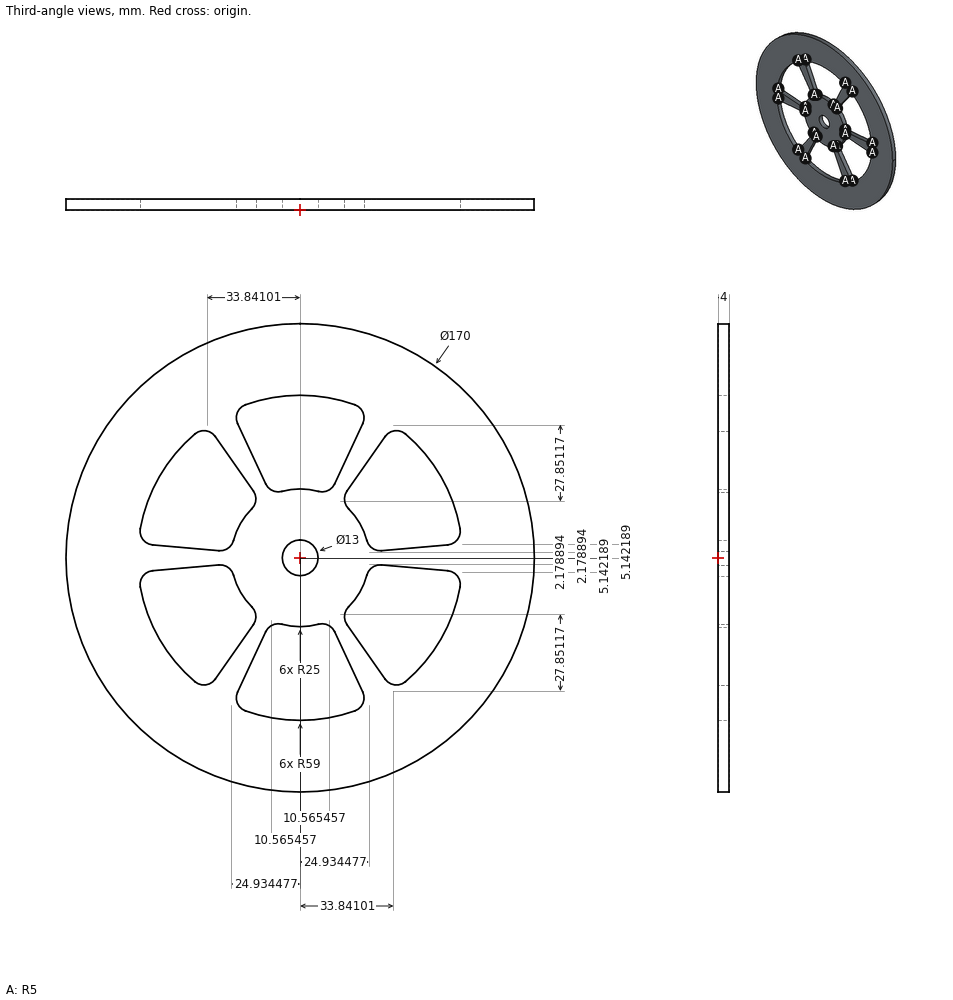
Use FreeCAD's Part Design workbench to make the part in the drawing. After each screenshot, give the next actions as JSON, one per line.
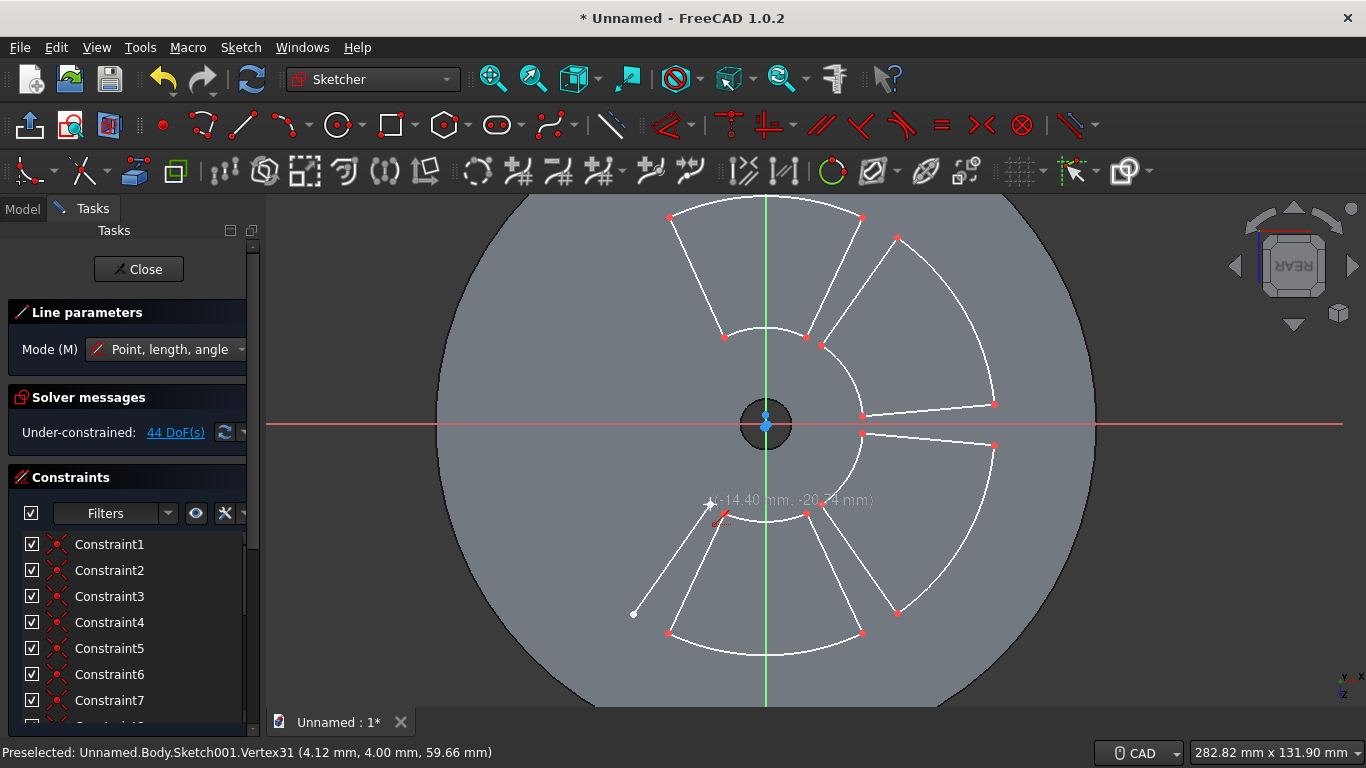
{"action": "scroll", "coordinate": [669, 433], "scroll_direction": "up", "scroll_amount": 4}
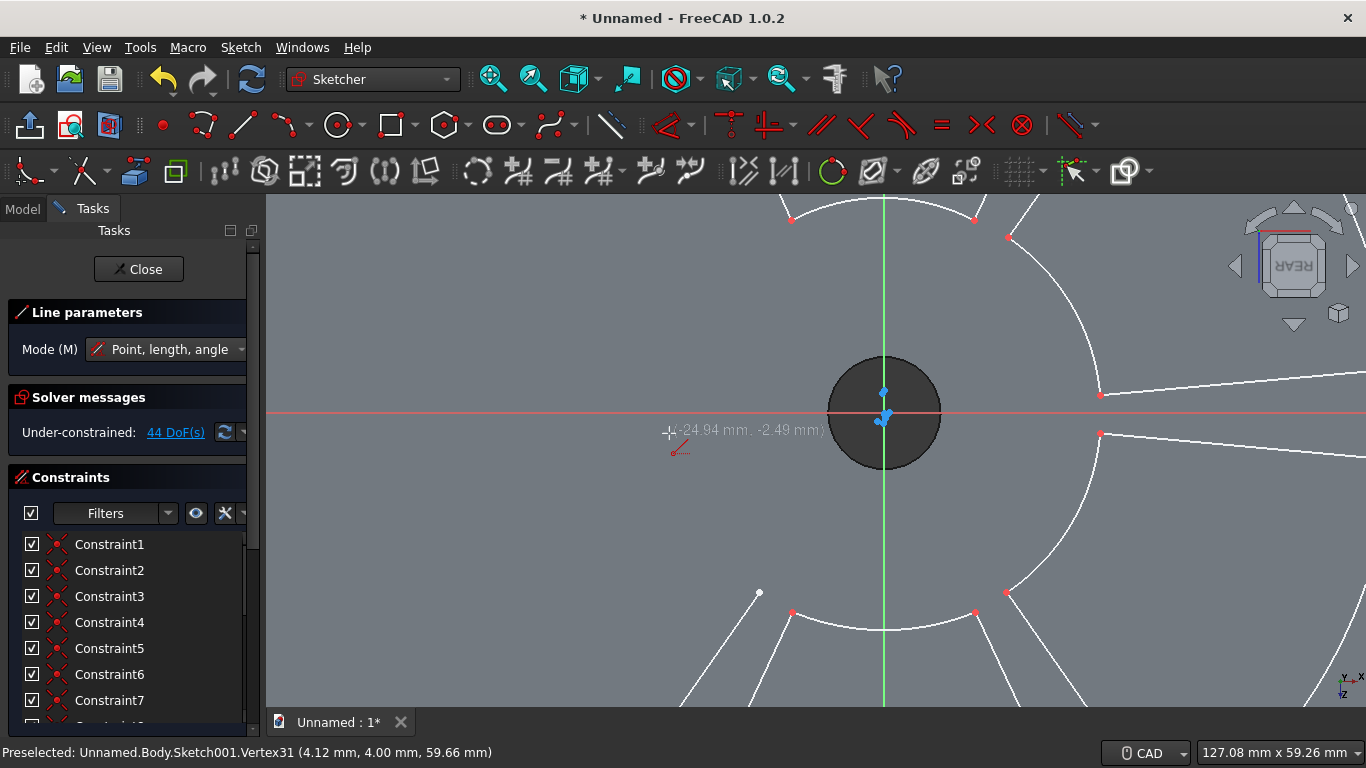
{"action": "left_click", "coordinate": [669, 432]}
{"action": "left_click", "coordinate": [376, 458]}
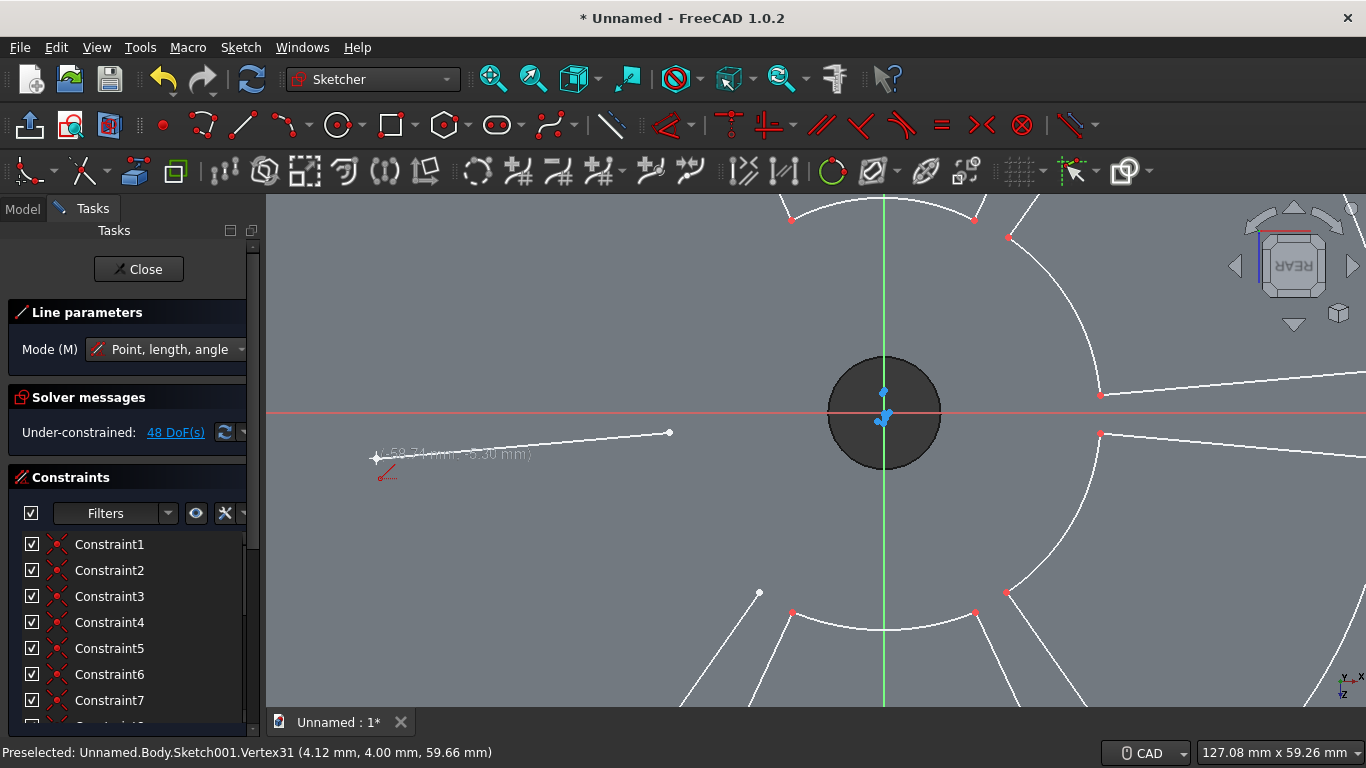
{"action": "left_click", "coordinate": [284, 126]}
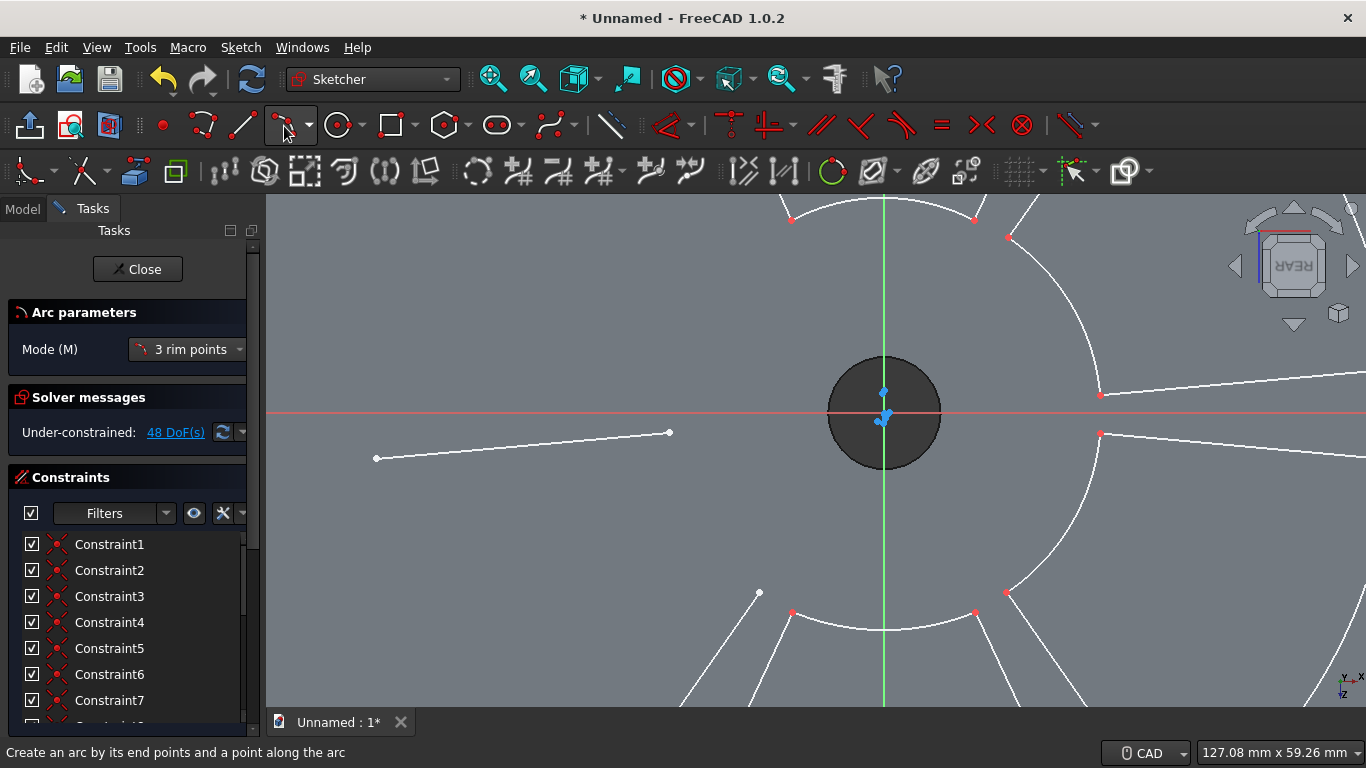
{"action": "left_click", "coordinate": [760, 593]}
{"action": "left_click", "coordinate": [669, 433]}
{"action": "left_click", "coordinate": [697, 521]}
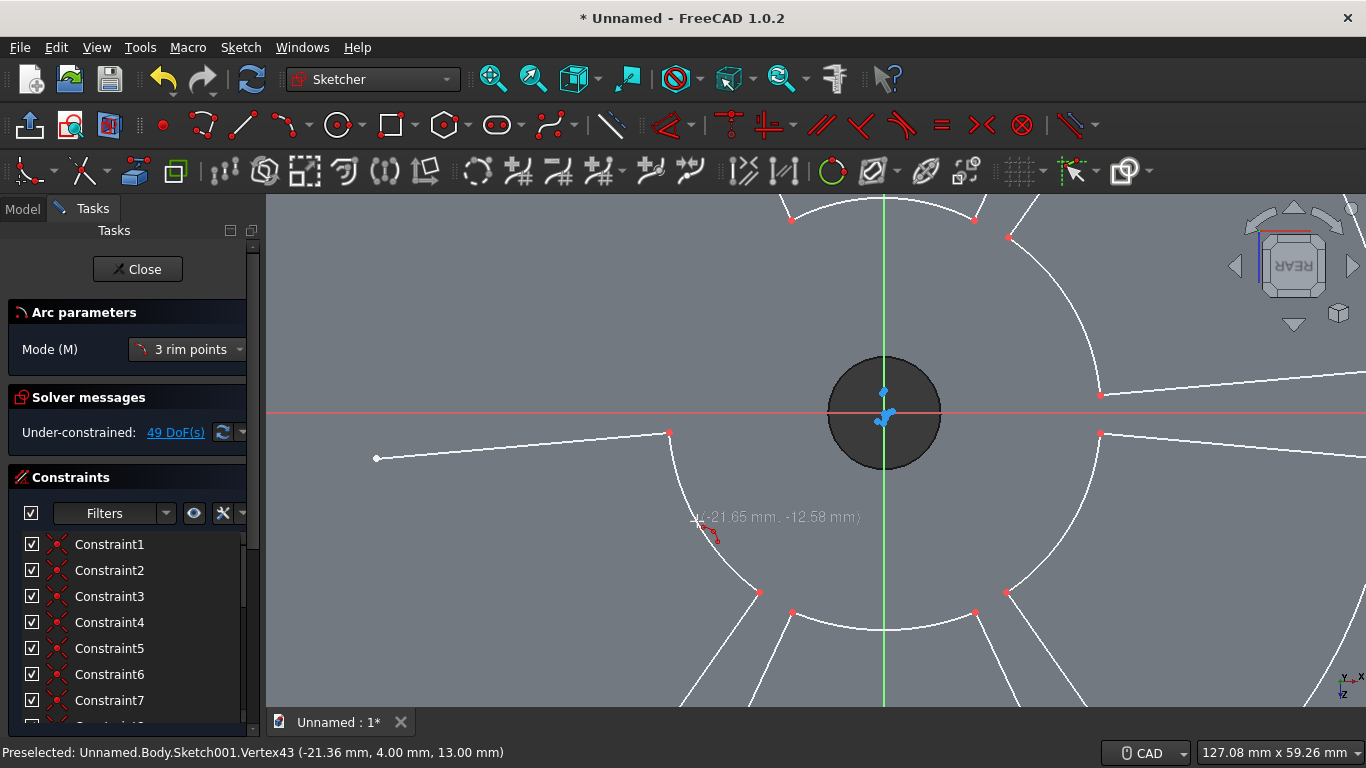
{"action": "left_click", "coordinate": [376, 459]}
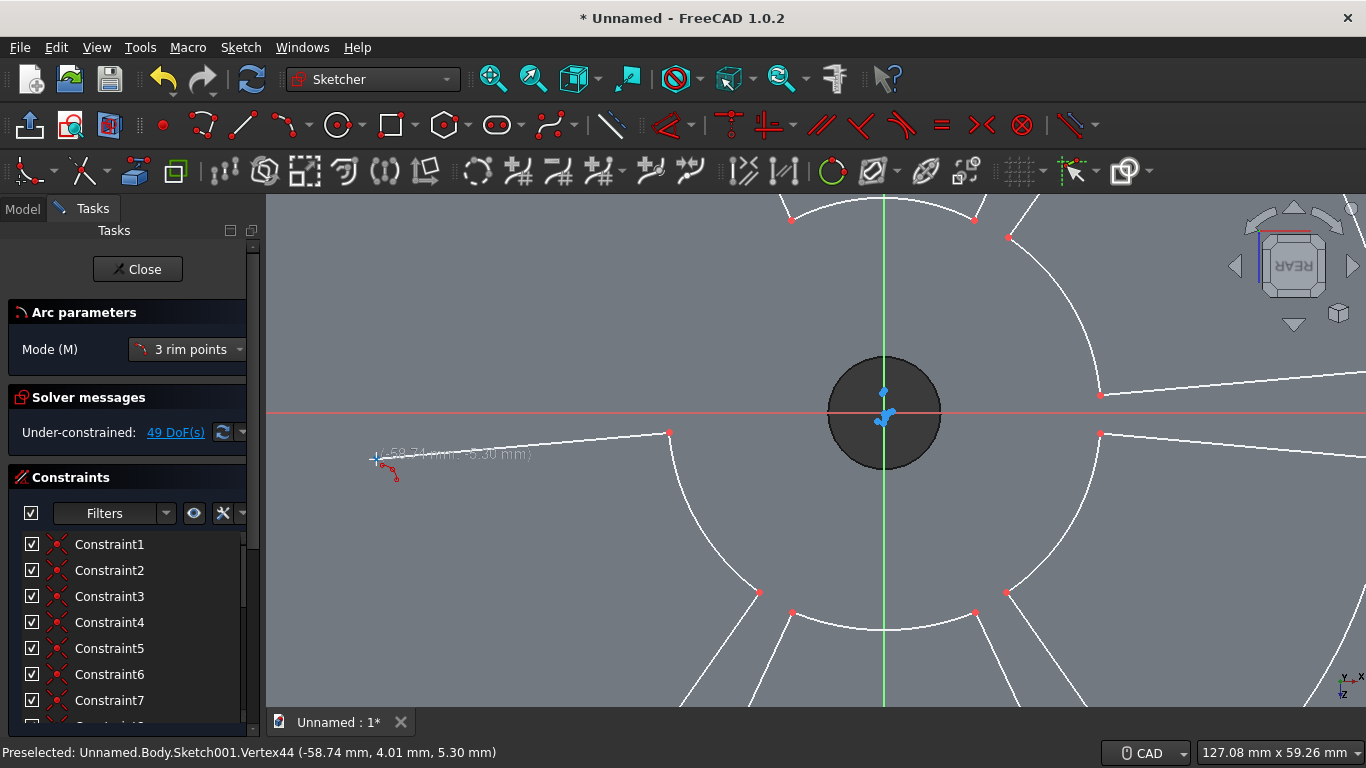
{"action": "scroll", "coordinate": [688, 467], "scroll_direction": "down", "scroll_amount": 6}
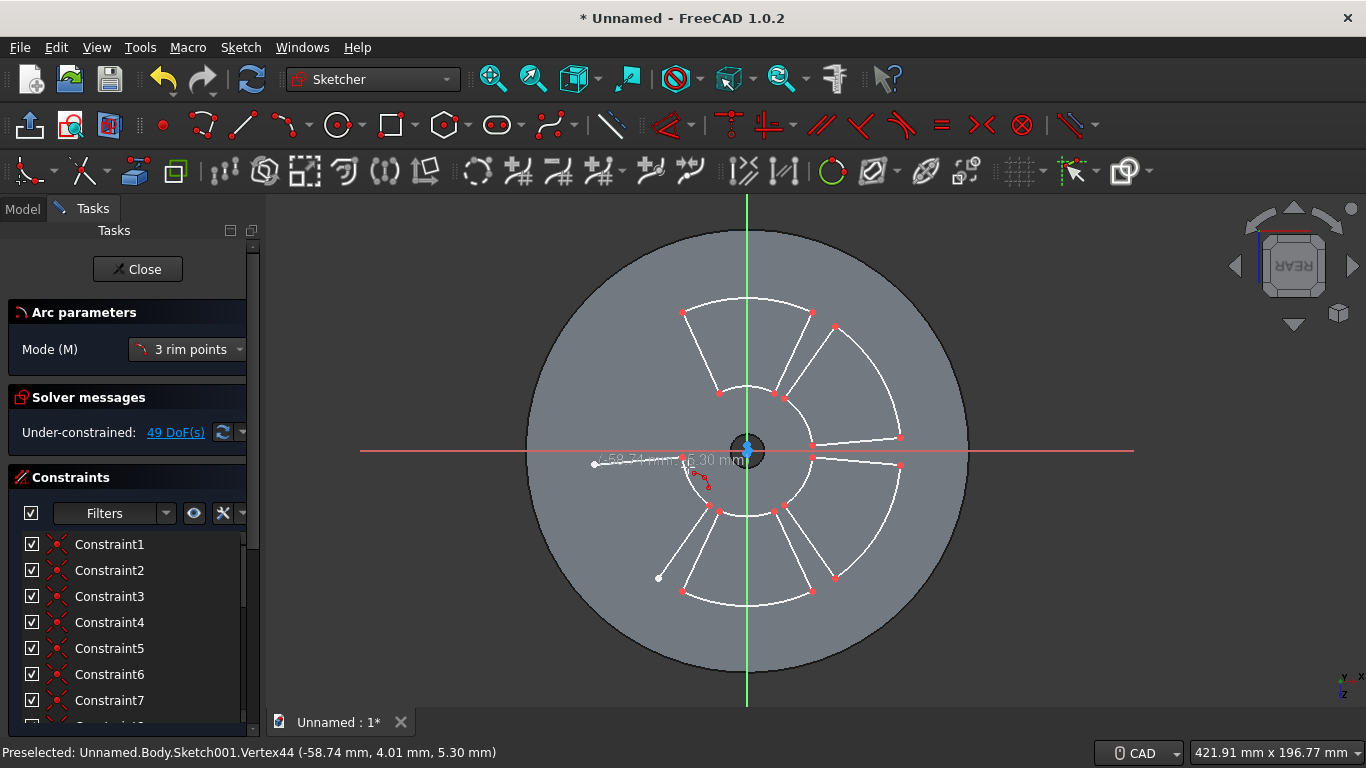
{"action": "left_click", "coordinate": [659, 578]}
{"action": "left_click", "coordinate": [614, 528]}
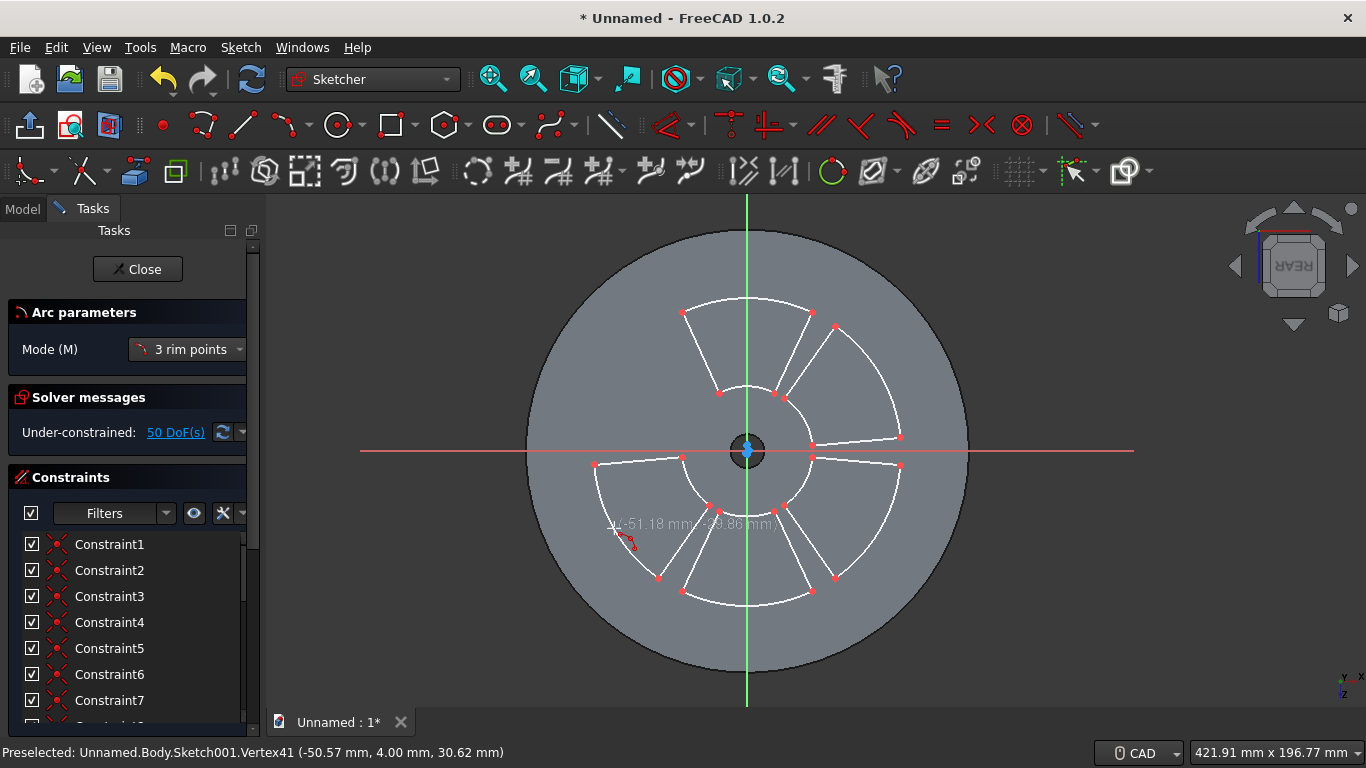
{"action": "left_click", "coordinate": [244, 126]}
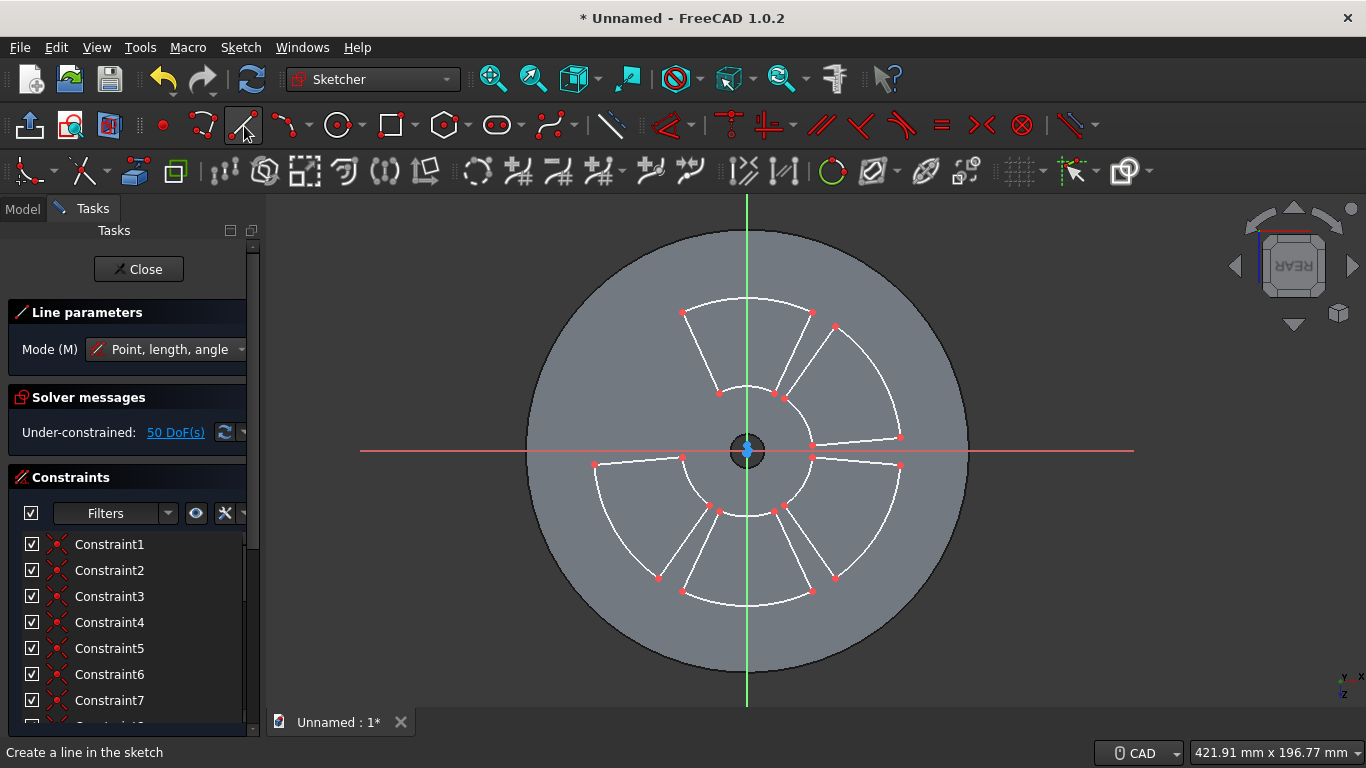
{"action": "left_click", "coordinate": [594, 438]}